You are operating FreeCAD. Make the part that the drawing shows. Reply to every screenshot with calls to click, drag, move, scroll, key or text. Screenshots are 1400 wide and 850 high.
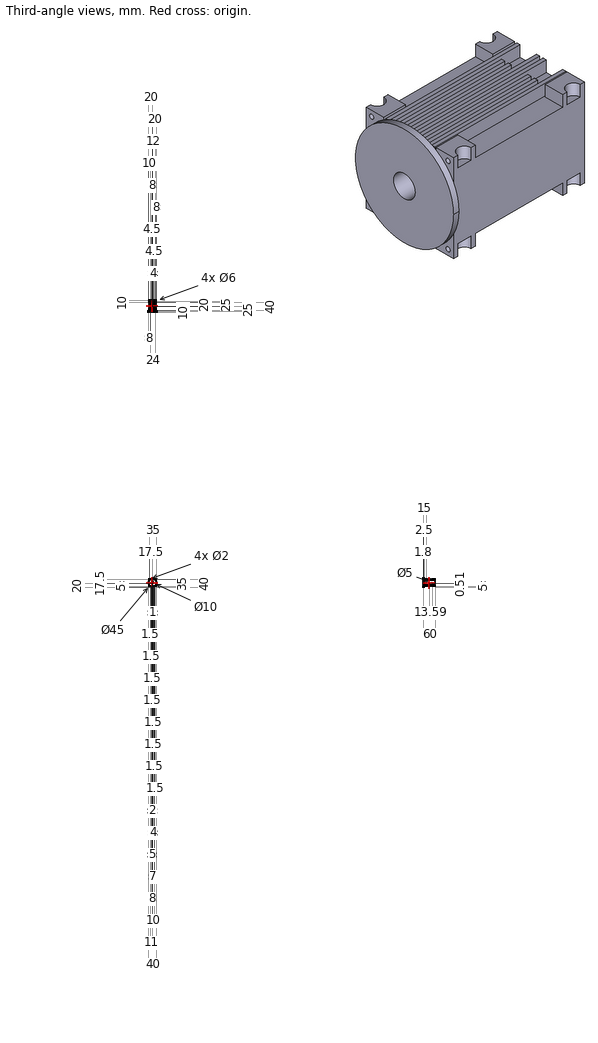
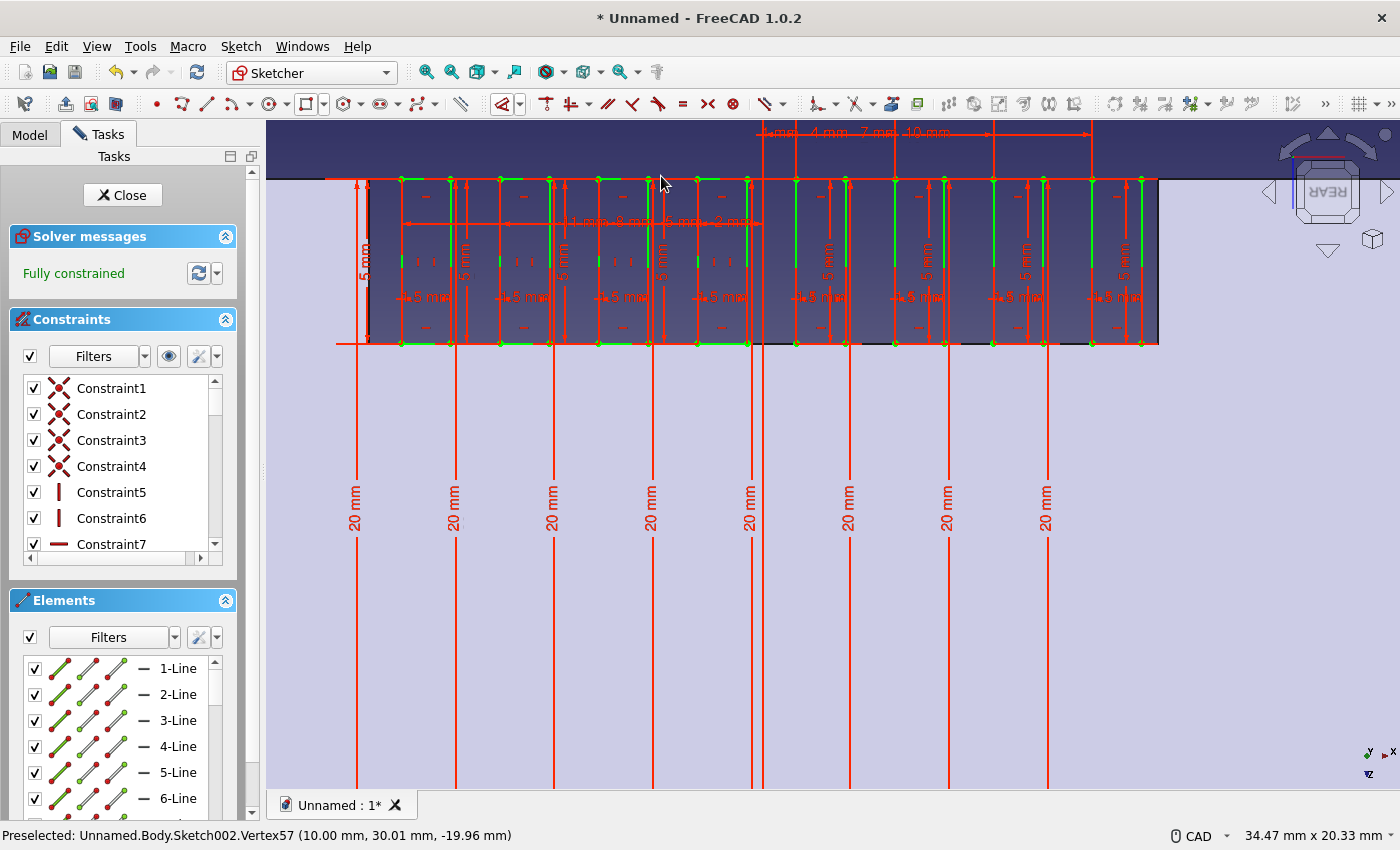
click(123, 195)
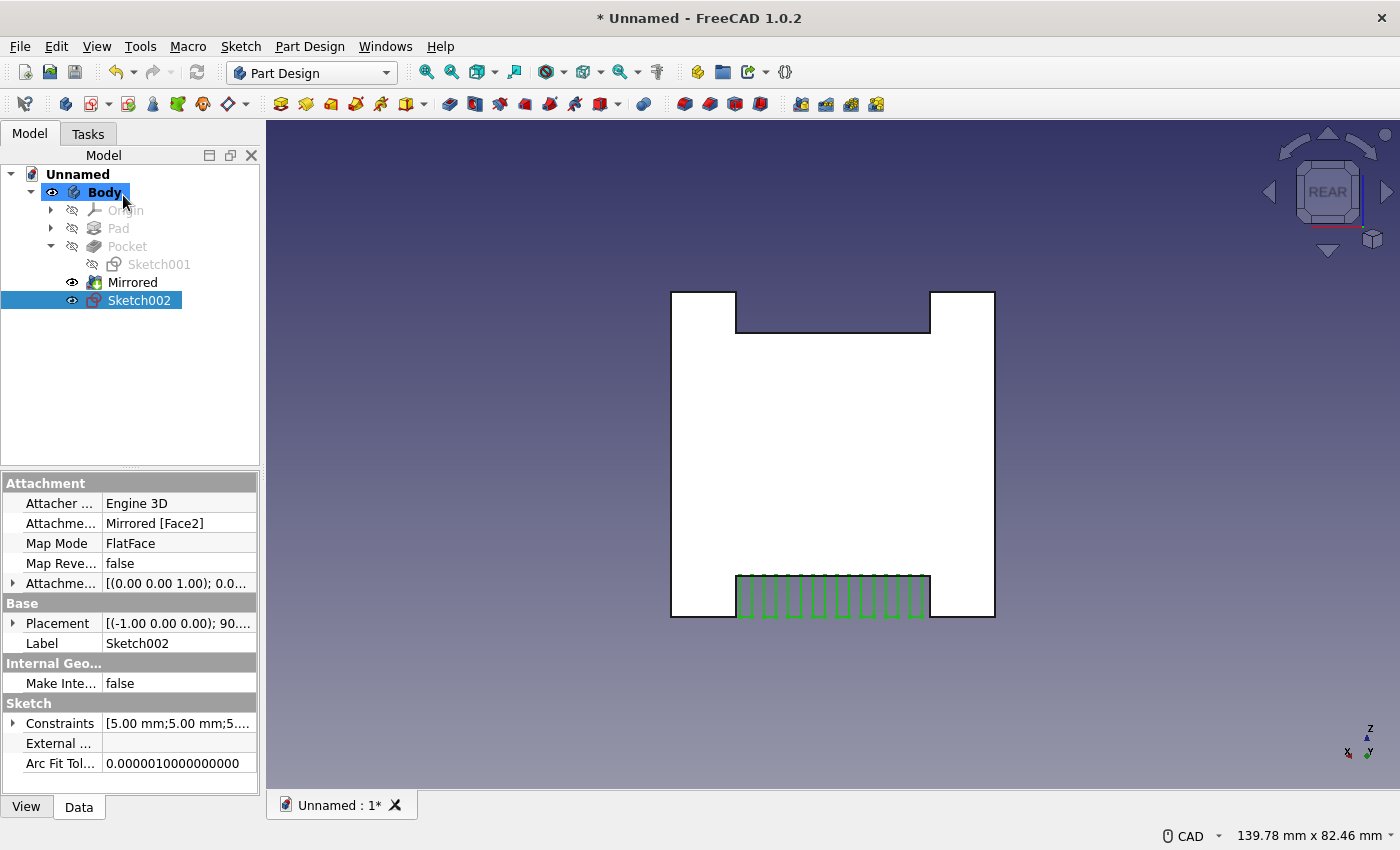
click(281, 104)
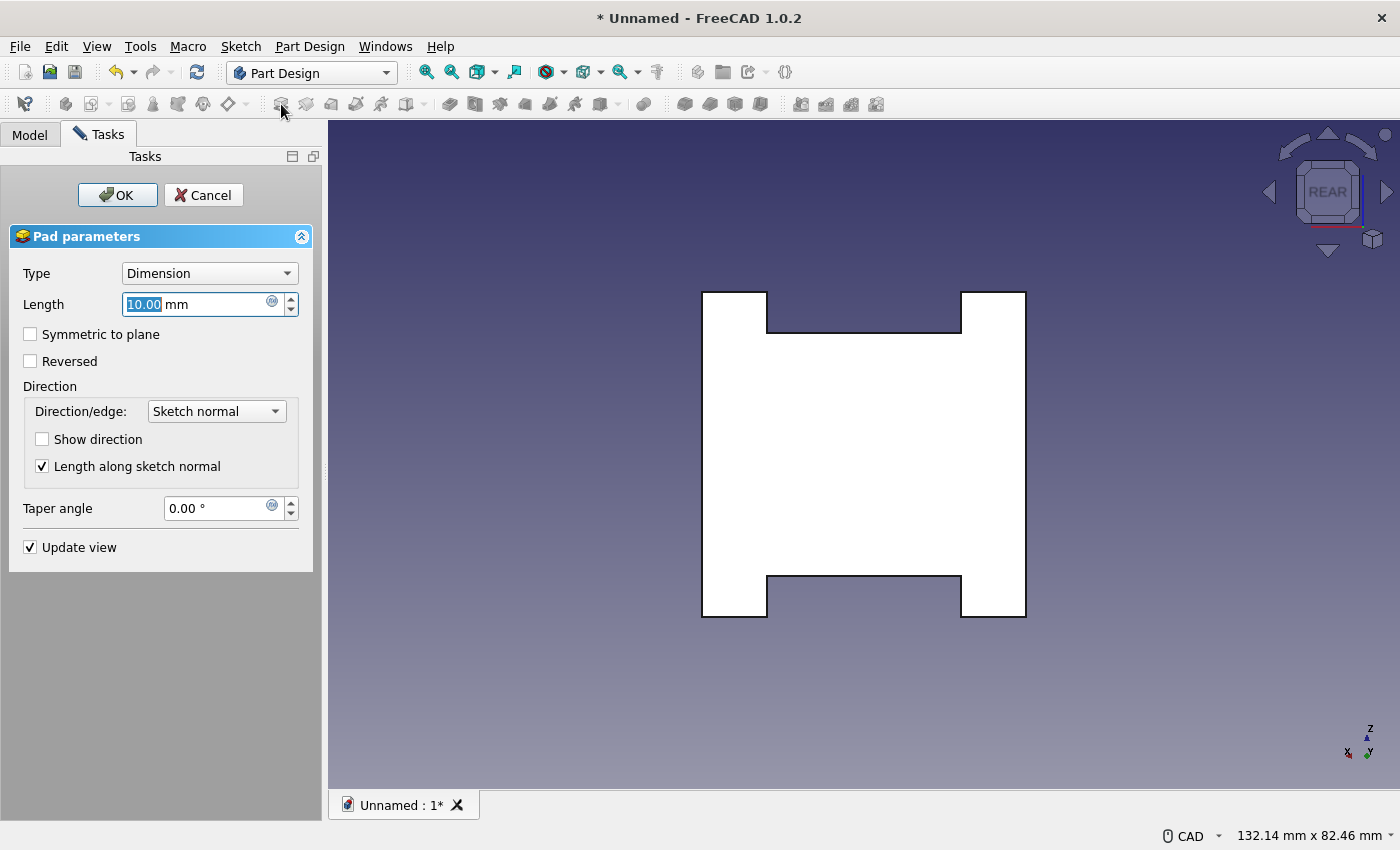
text(60)
key(Tab)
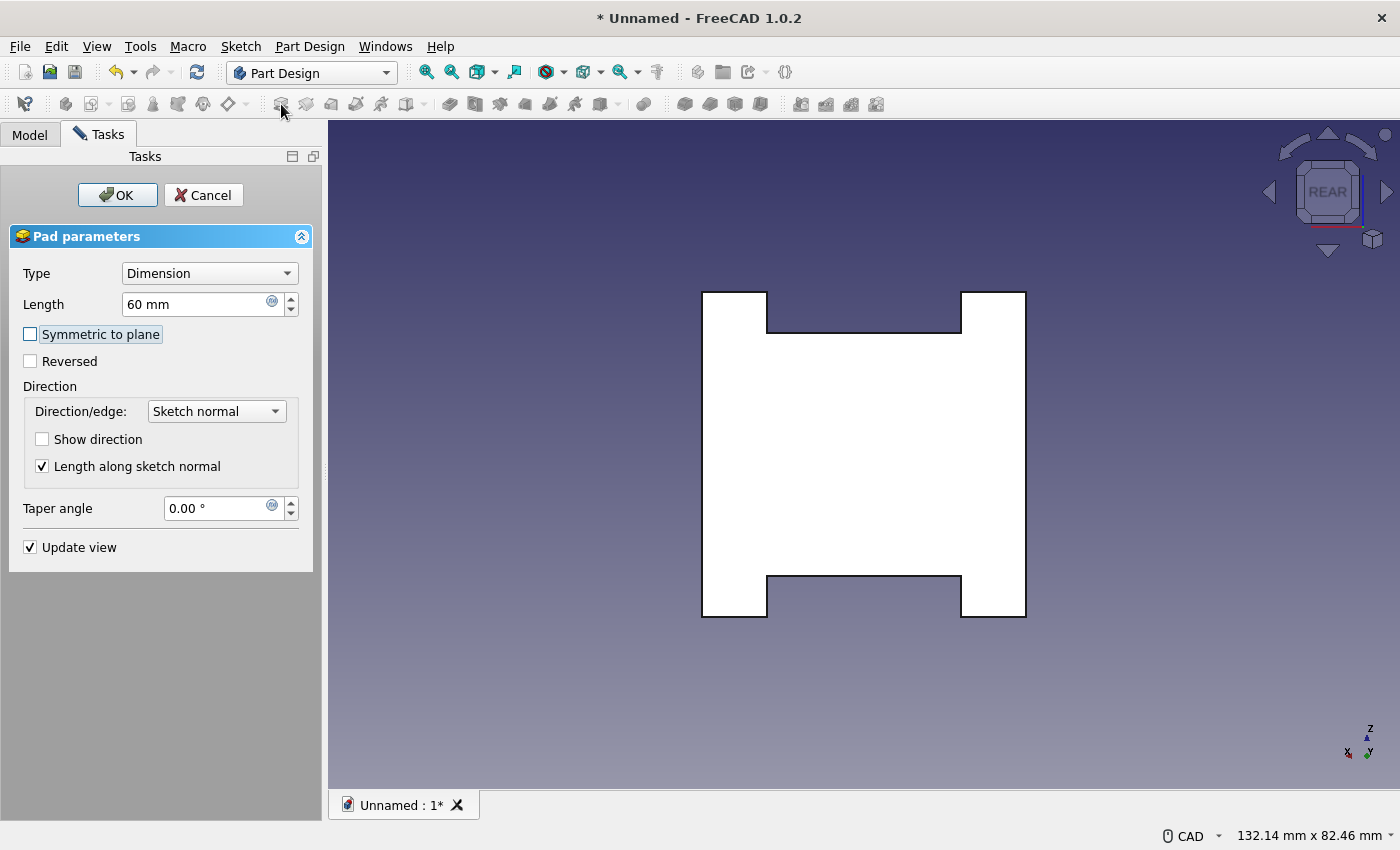
click(31, 361)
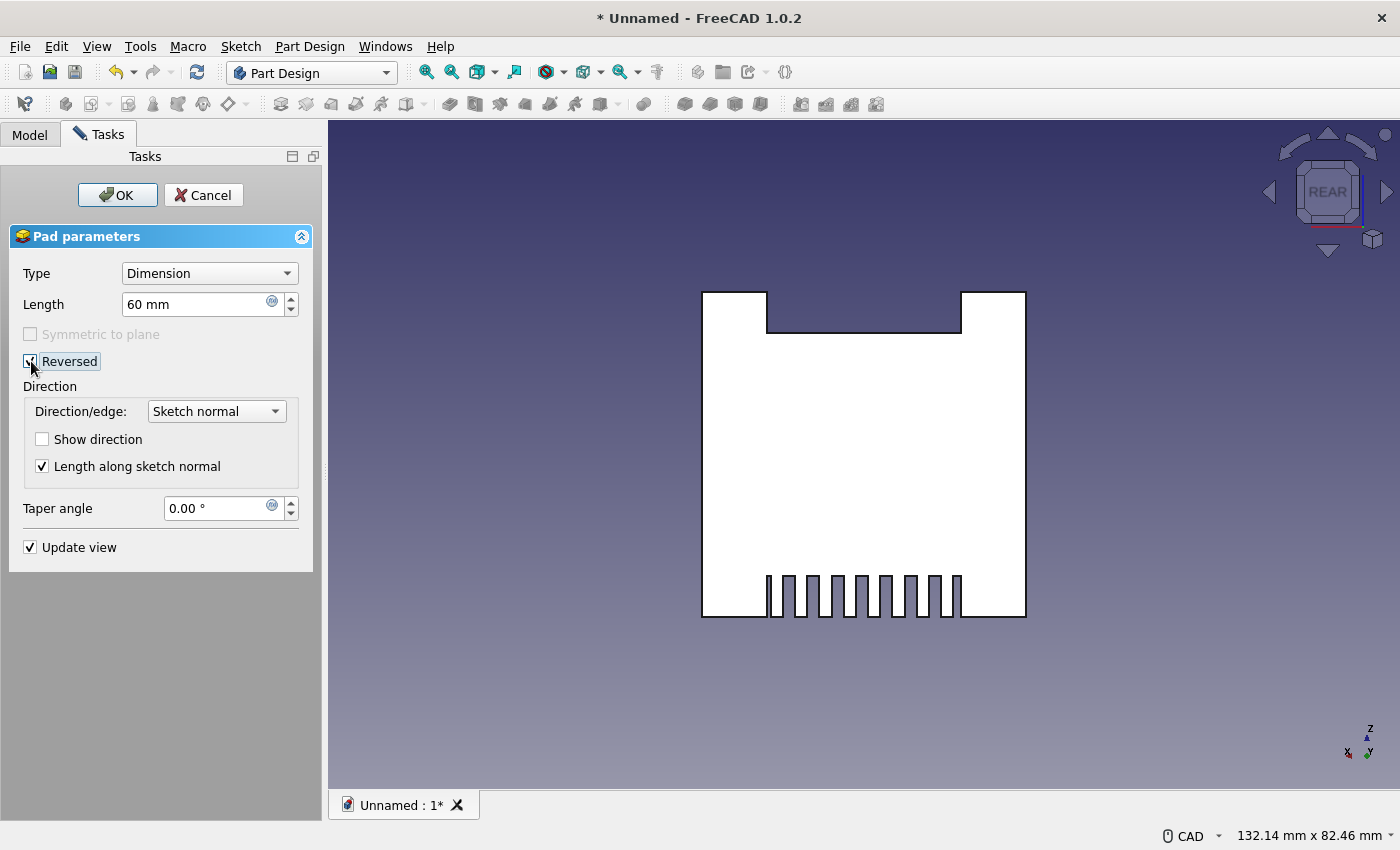
click(118, 195)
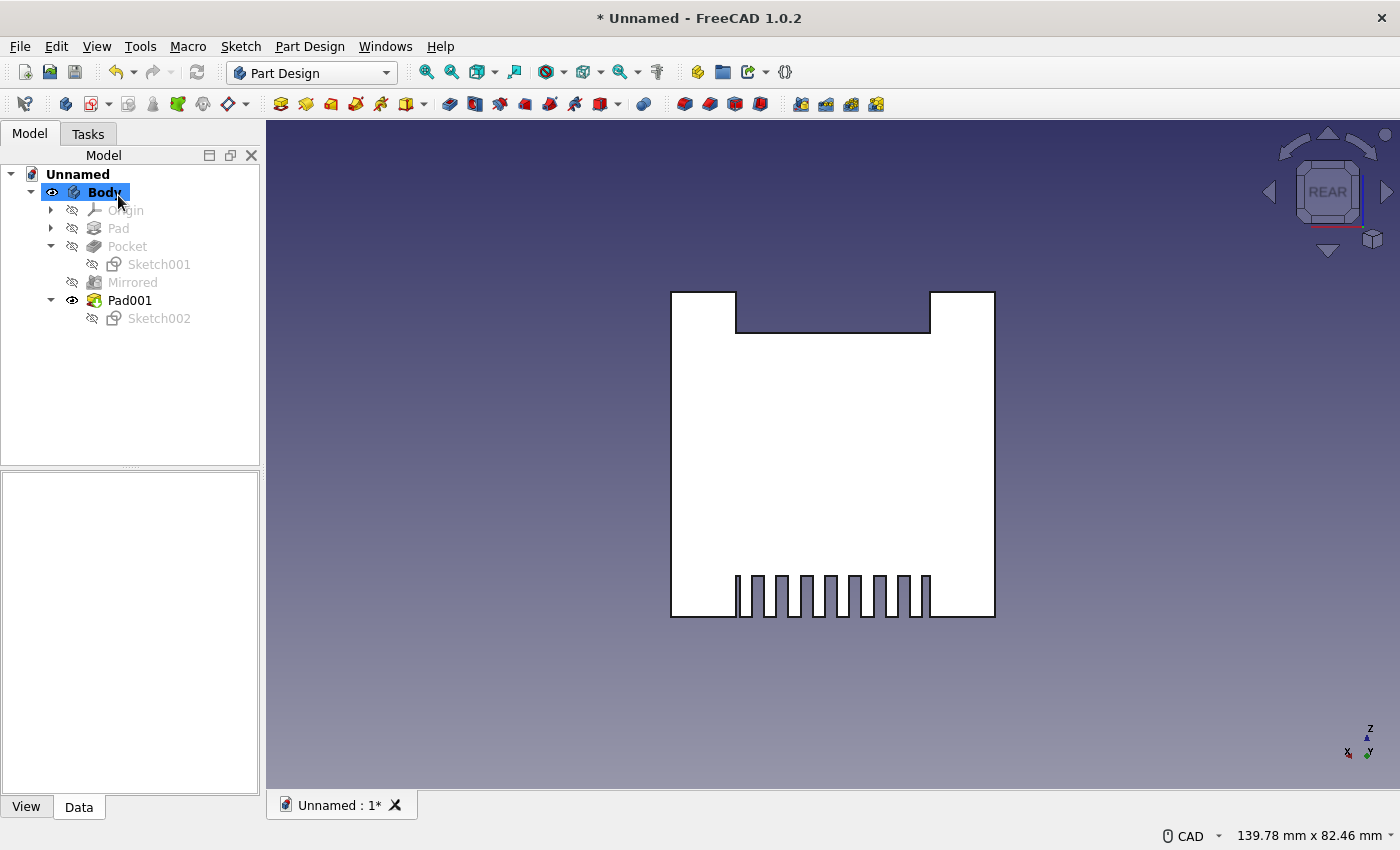
key(5)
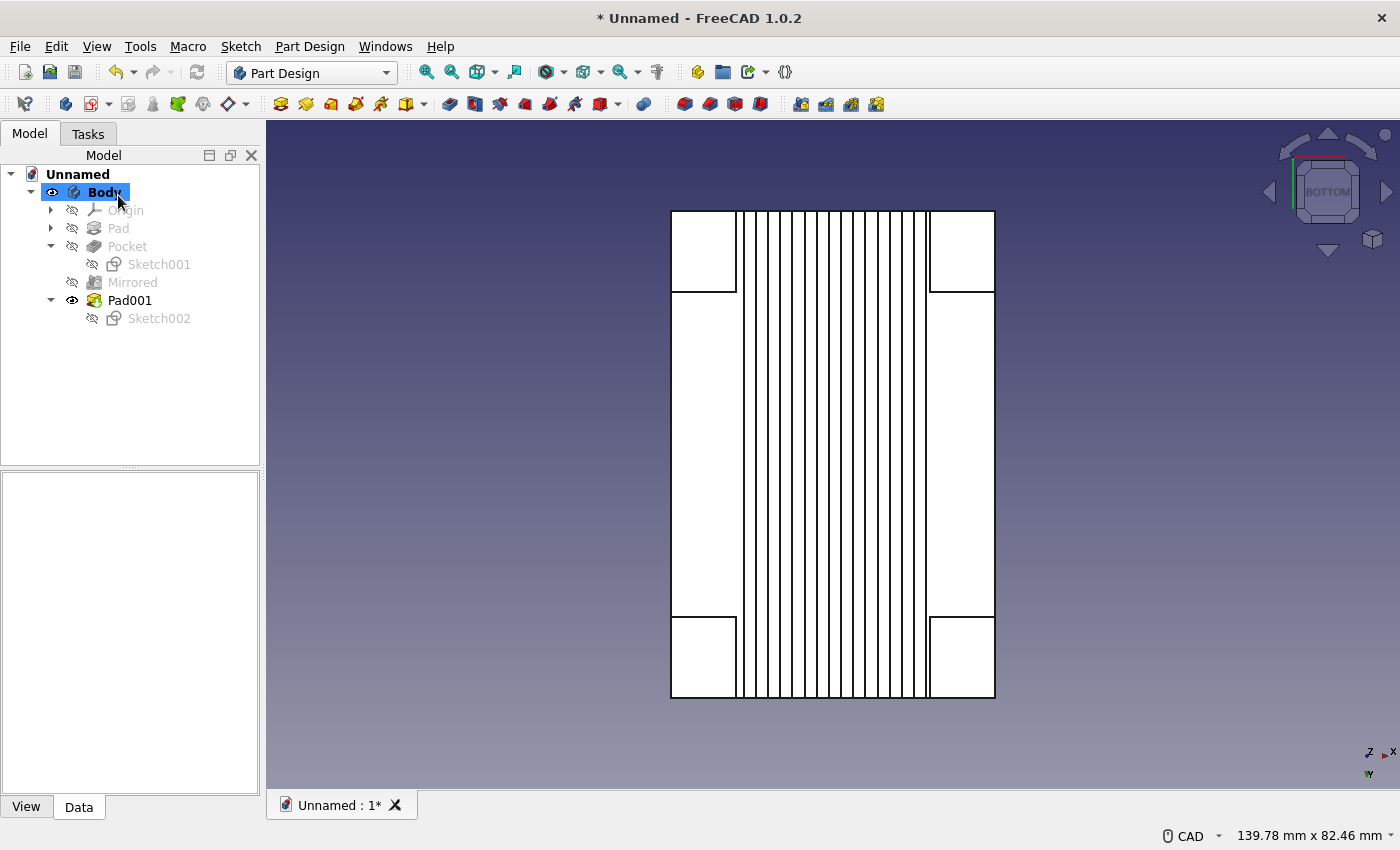
scroll(847, 662, up, 4)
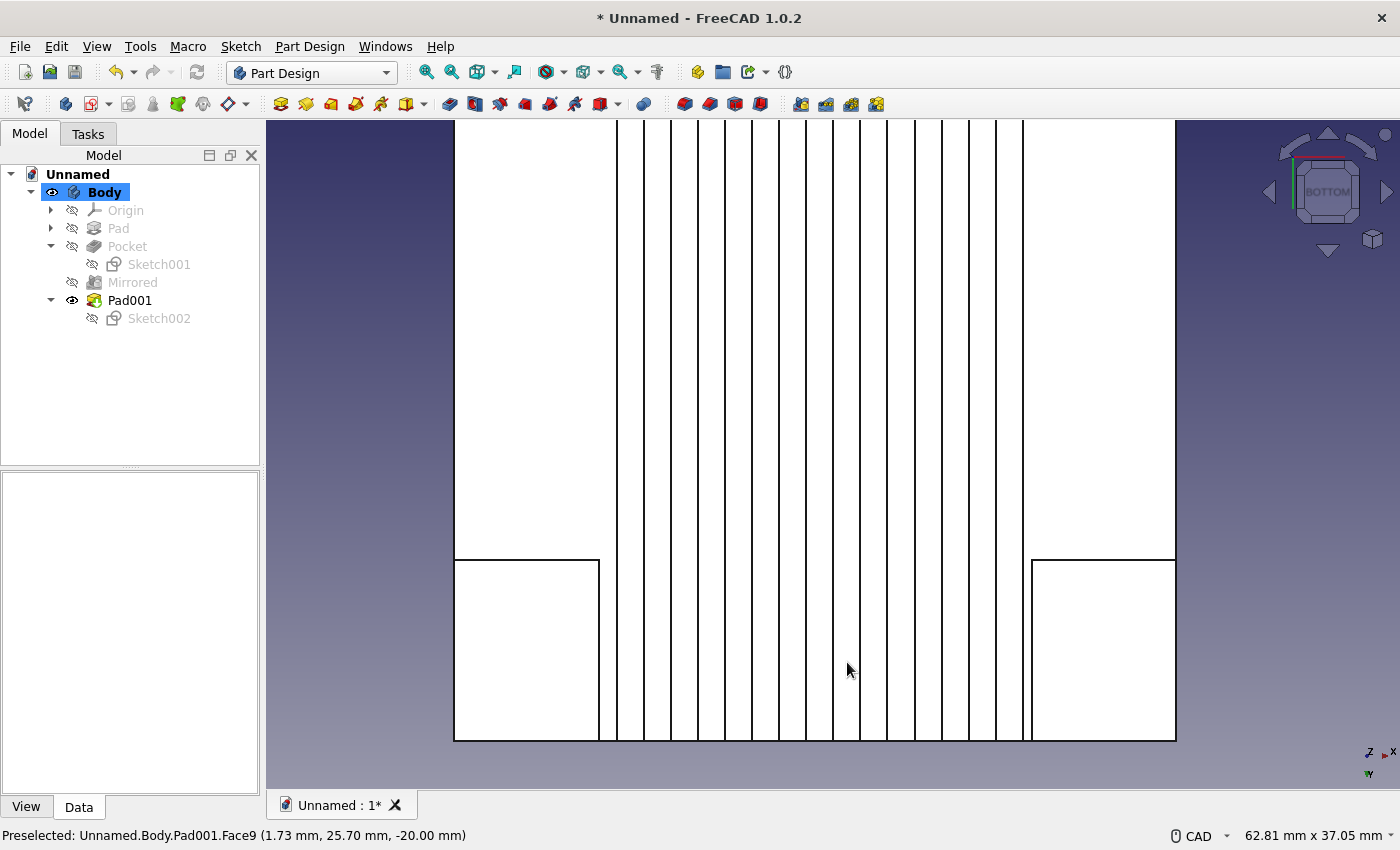
click(847, 662)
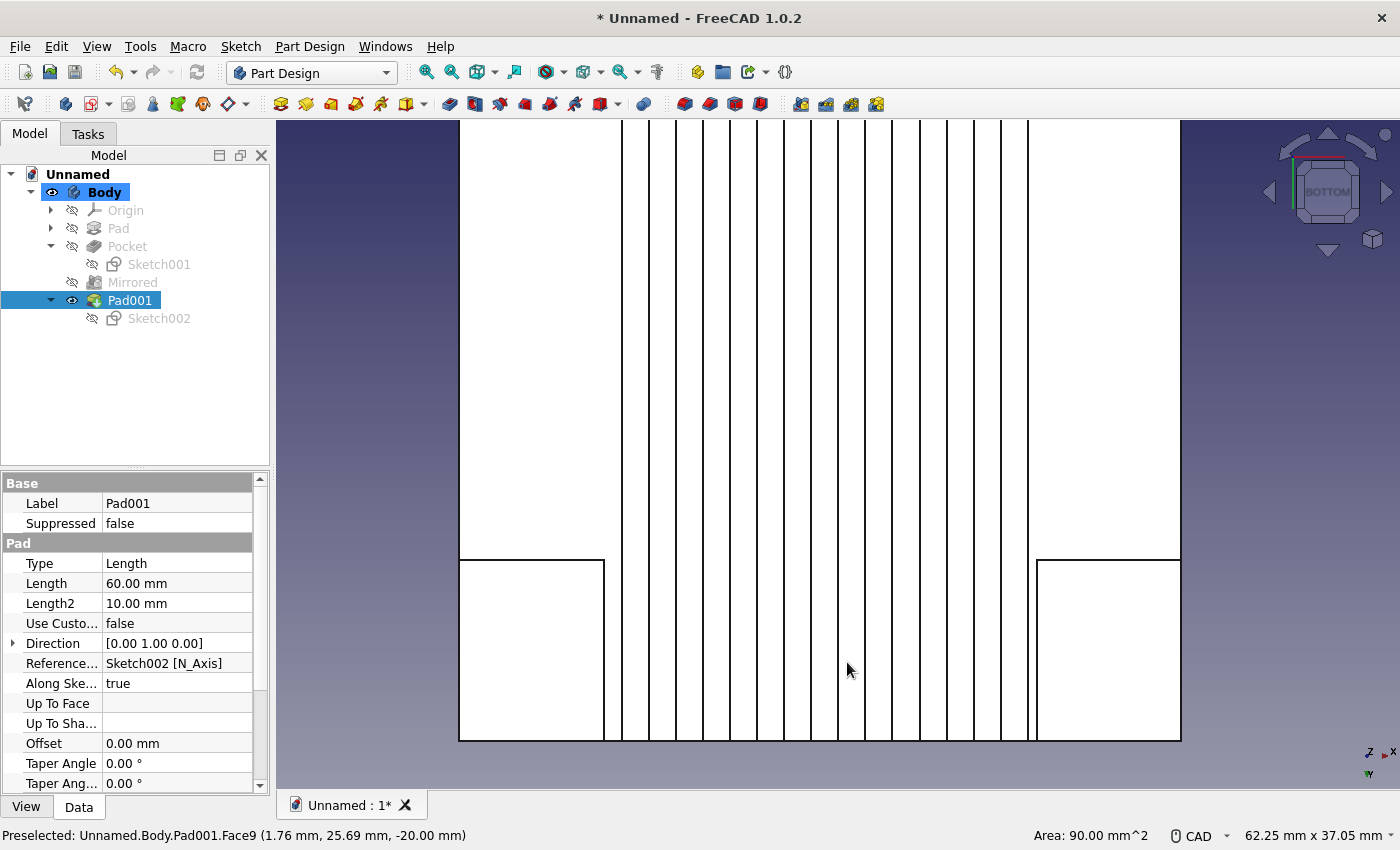
click(90, 104)